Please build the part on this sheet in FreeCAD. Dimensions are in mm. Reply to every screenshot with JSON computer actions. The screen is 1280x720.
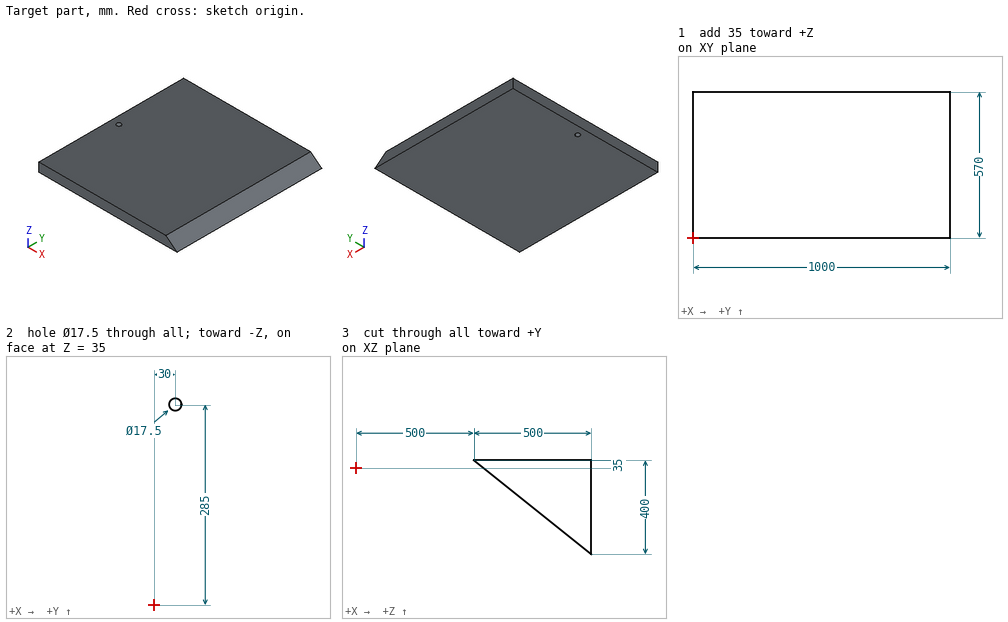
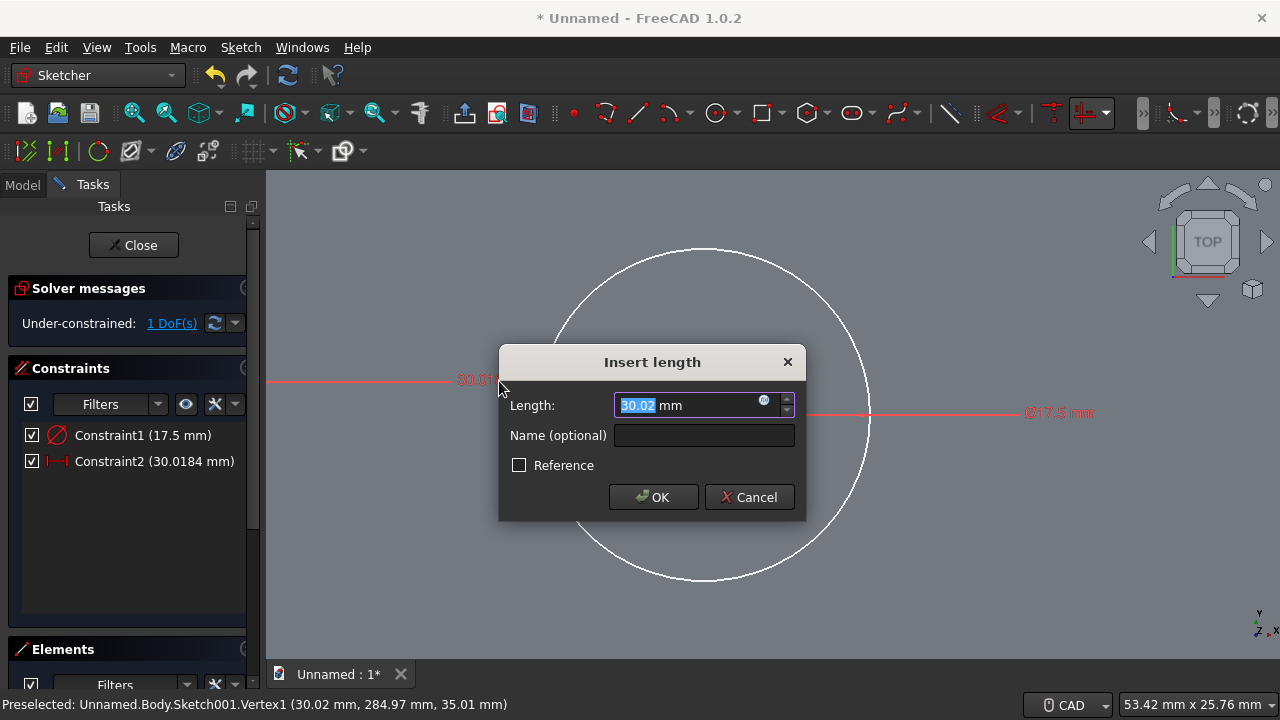
{"action": "type", "text": "30"}
{"action": "key", "text": "Return"}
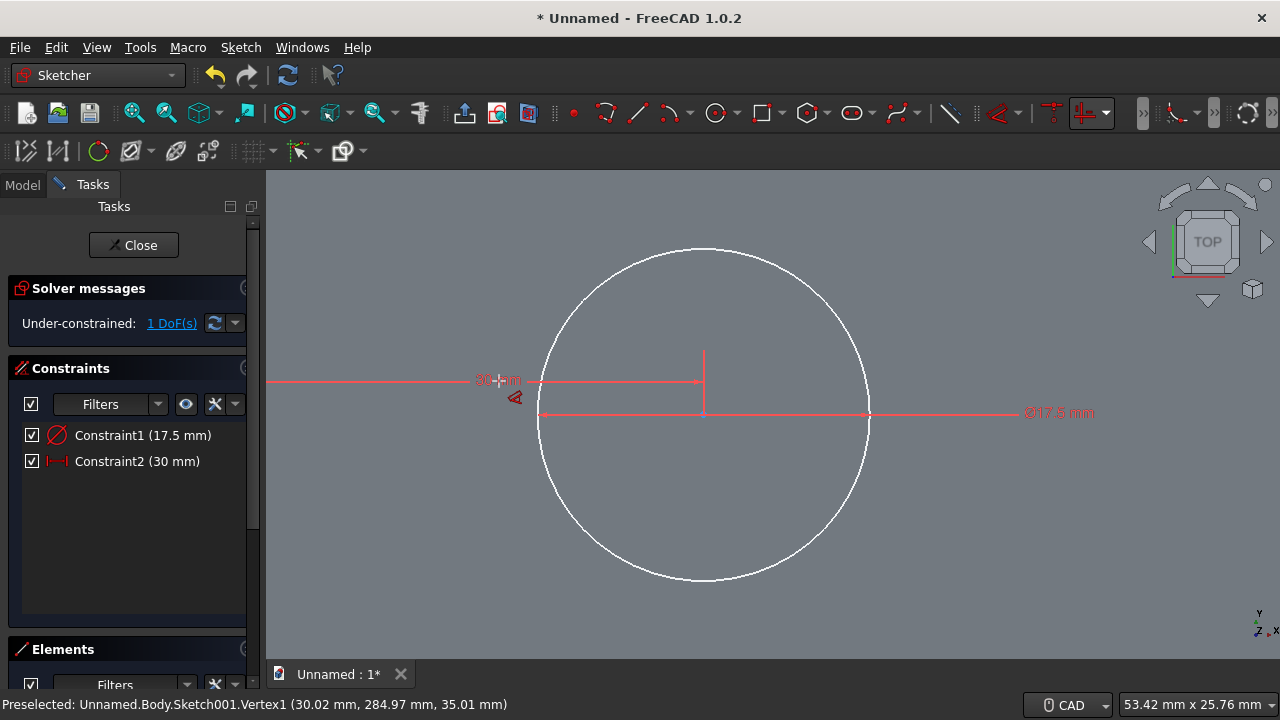
{"action": "left_click", "coordinate": [704, 415]}
{"action": "left_click", "coordinate": [738, 523]}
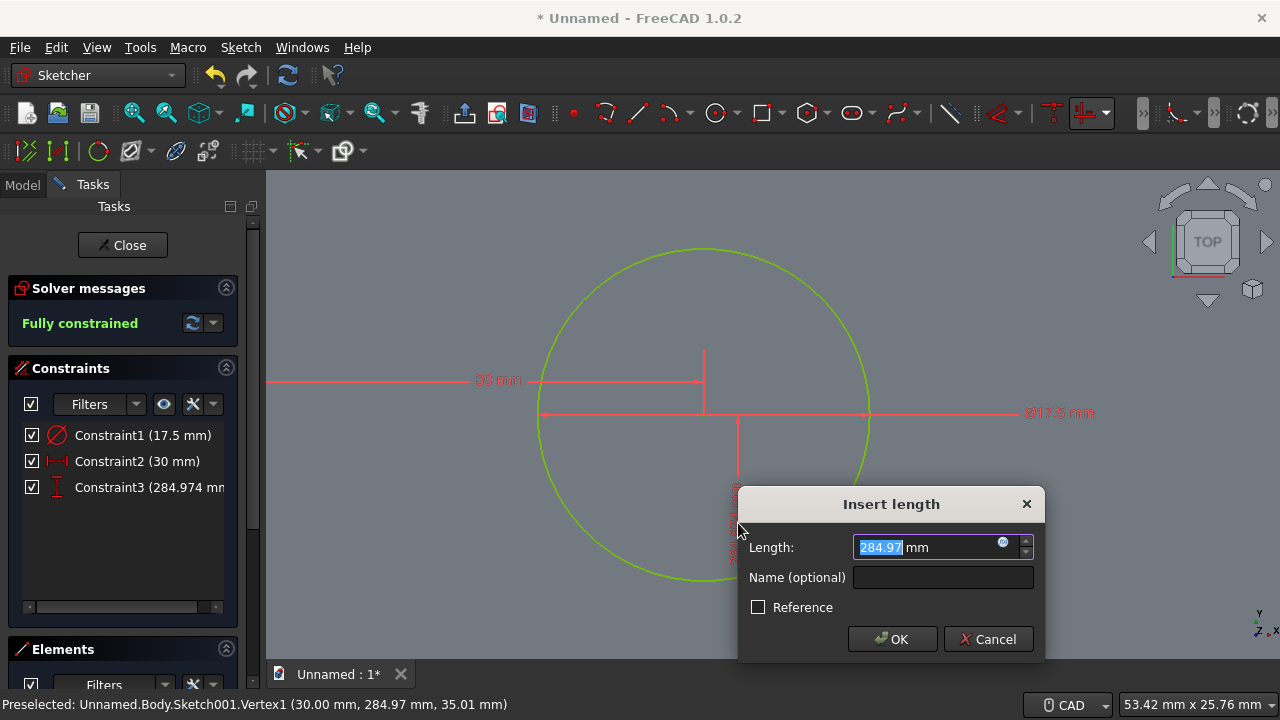
{"action": "type", "text": "285"}
{"action": "key", "text": "Return"}
{"action": "key", "text": "Escape"}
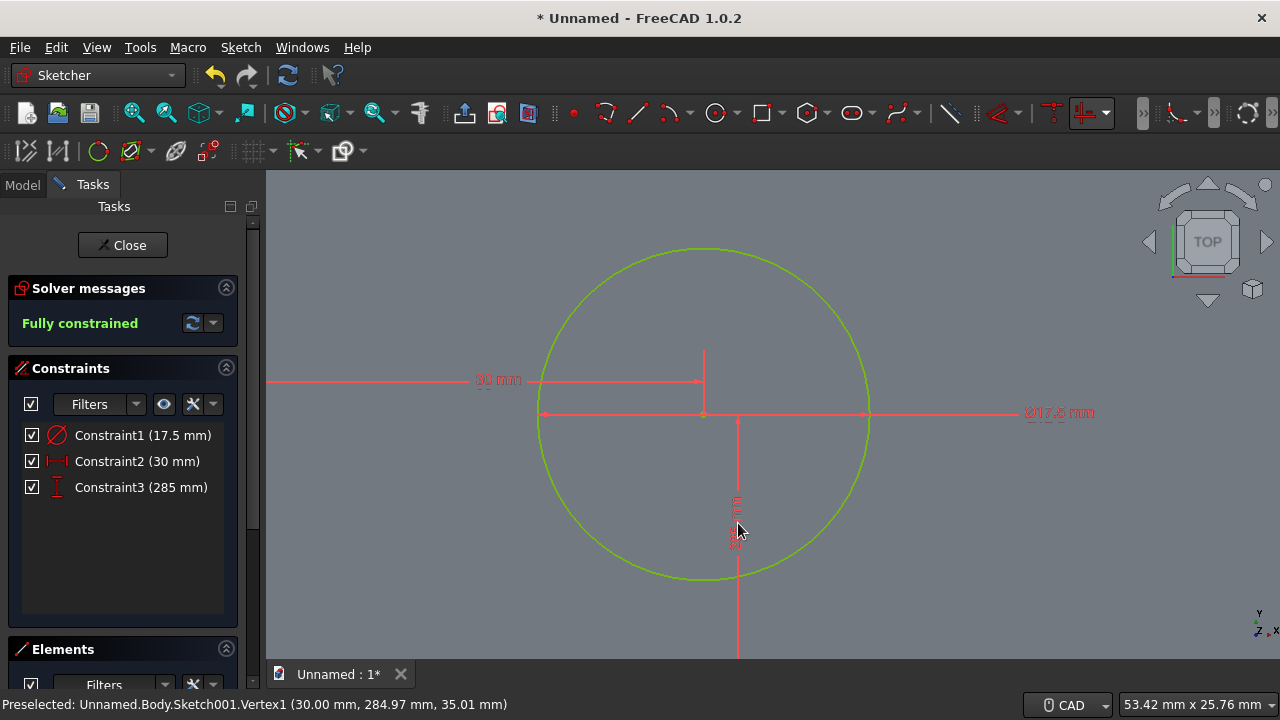
{"action": "left_click", "coordinate": [123, 245]}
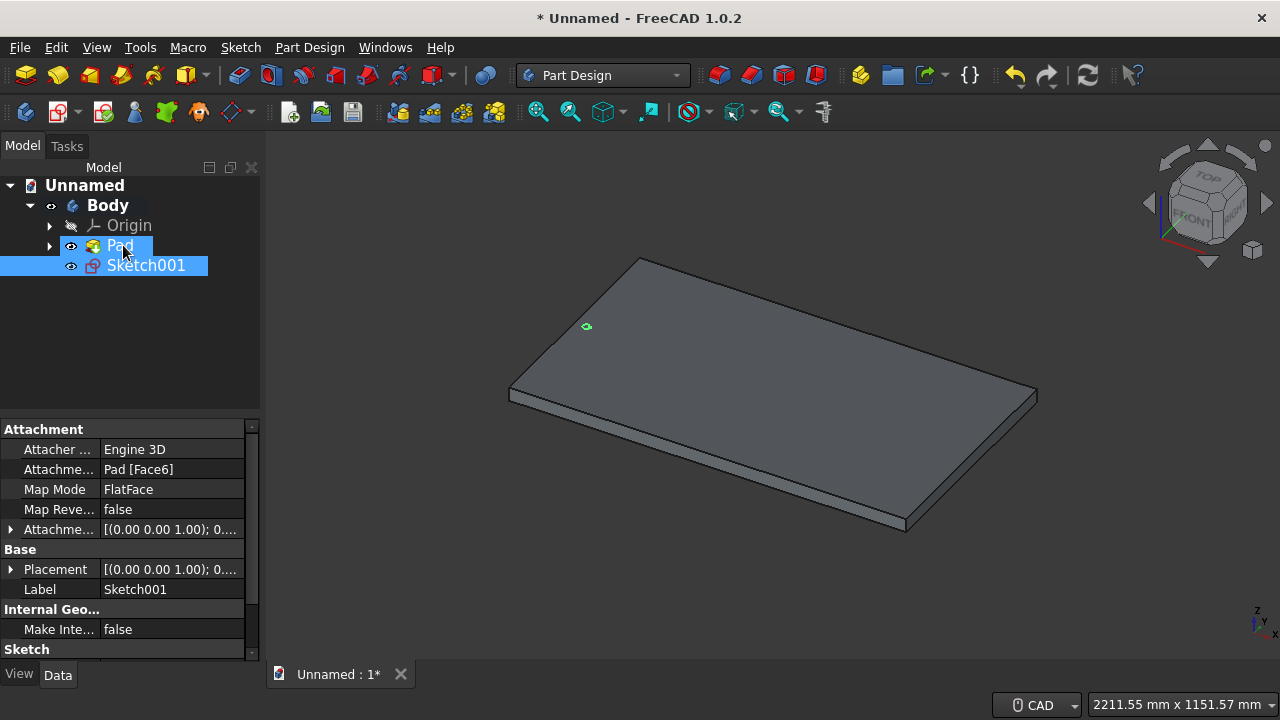
{"action": "left_click", "coordinate": [272, 76]}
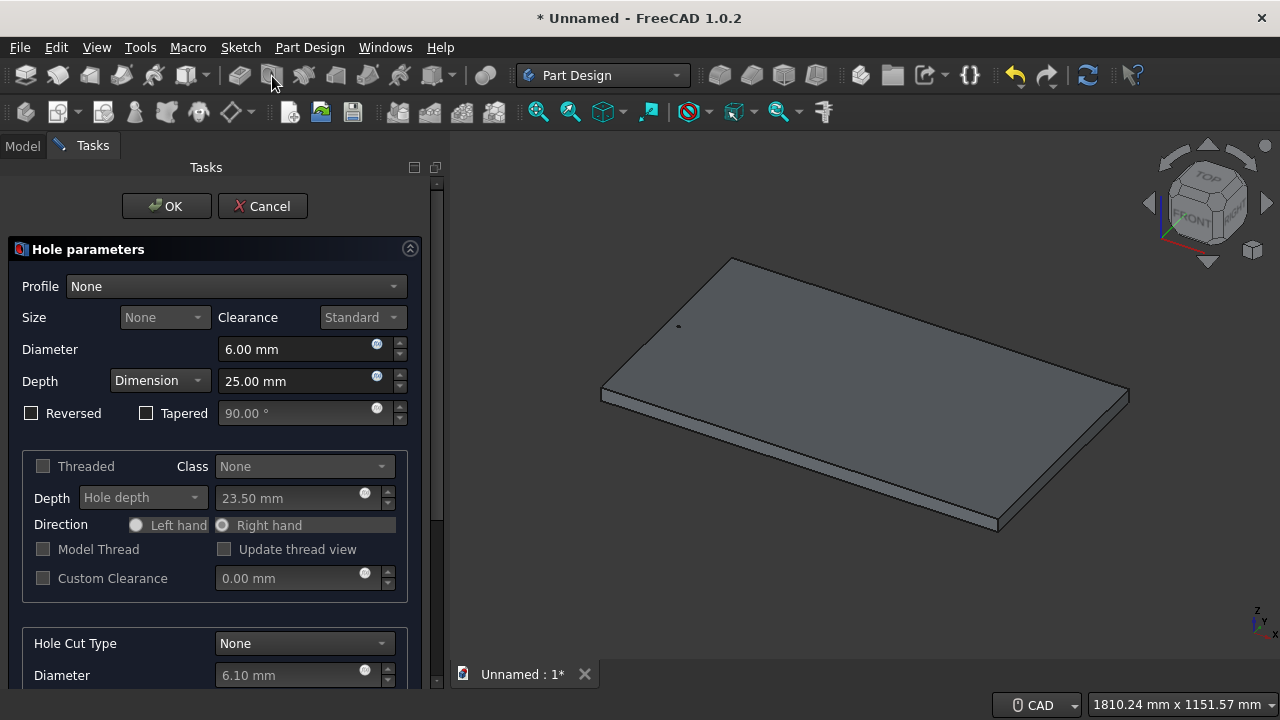
{"action": "triple_click", "coordinate": [305, 349]}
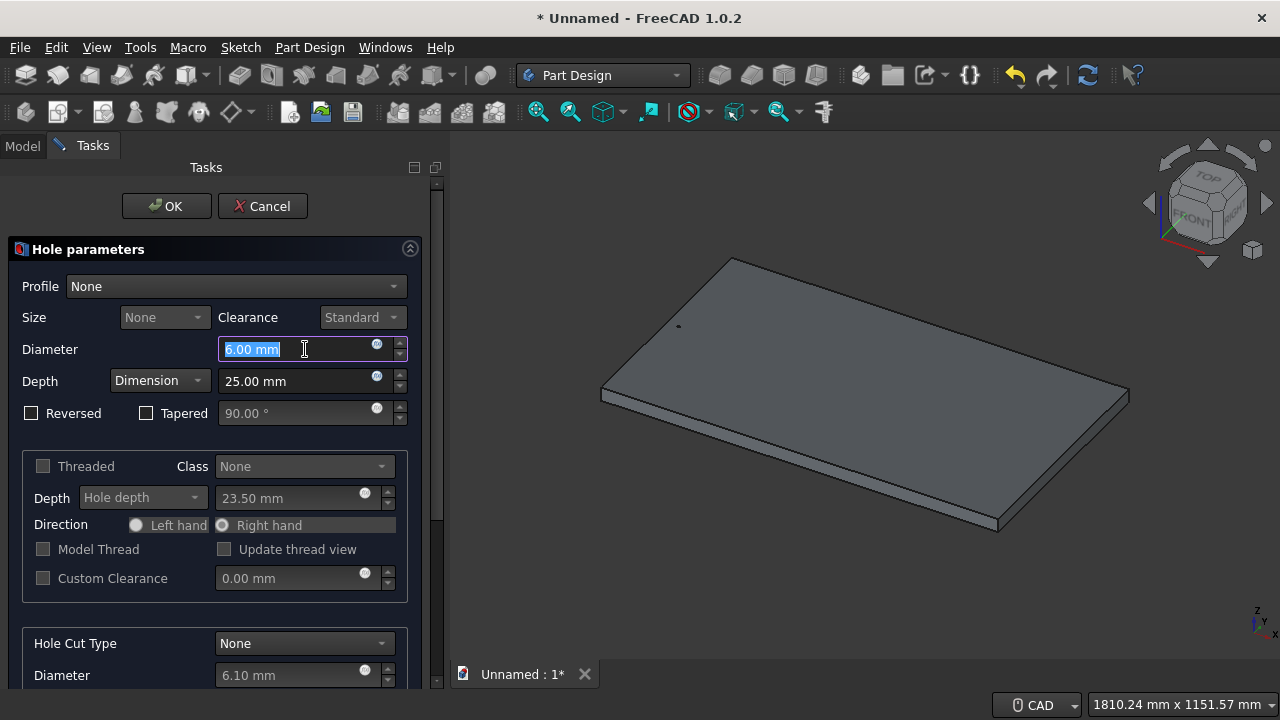
{"action": "type", "text": "17.5"}
{"action": "key", "text": "Tab"}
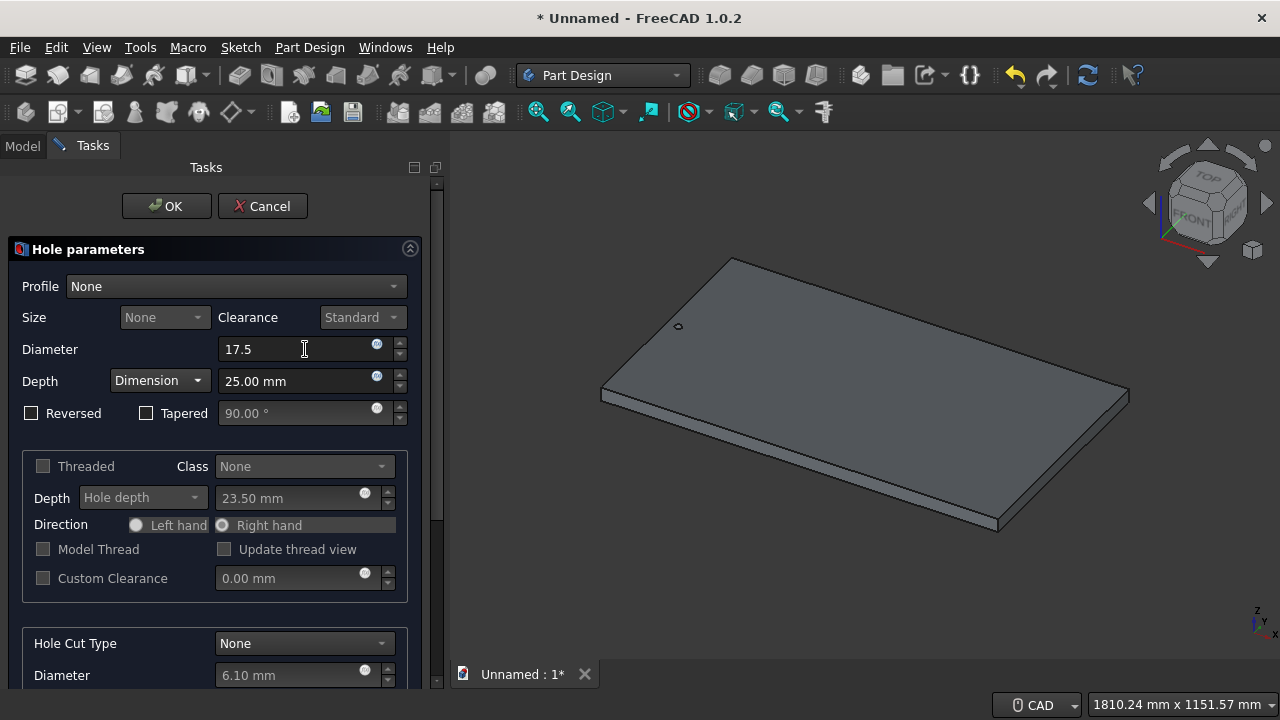
{"action": "left_click", "coordinate": [161, 380]}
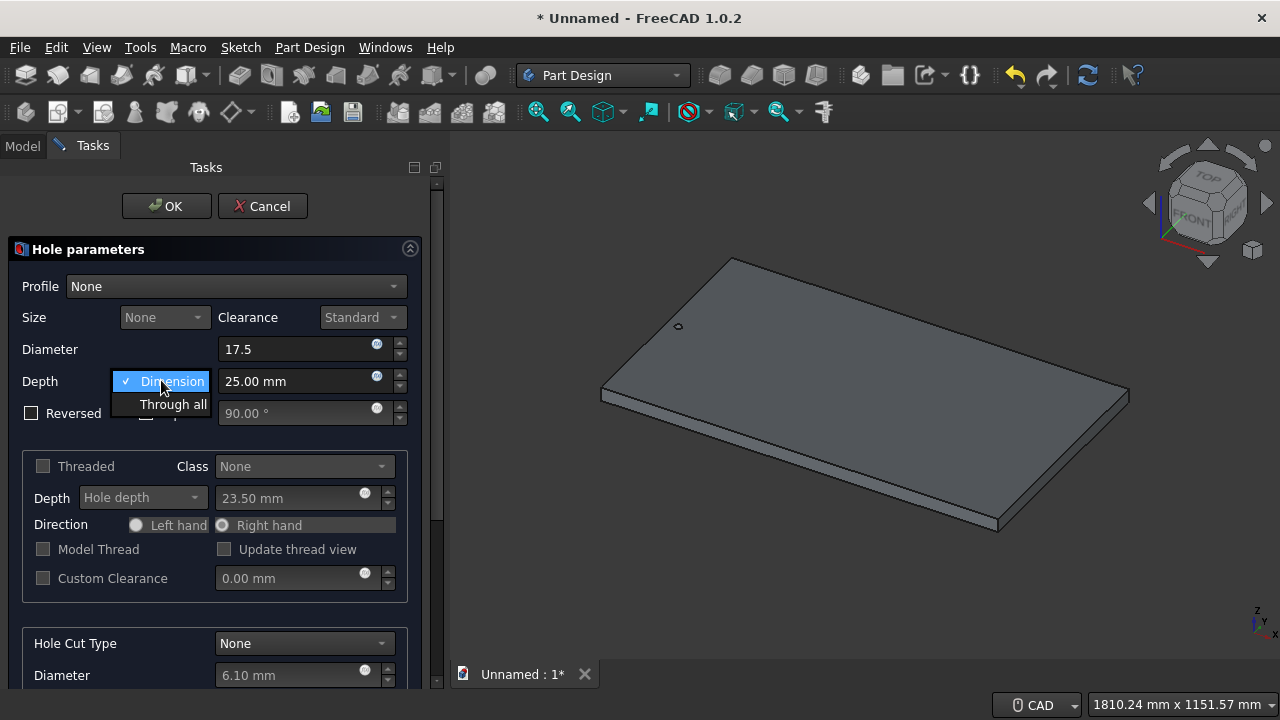
{"action": "left_click", "coordinate": [160, 404]}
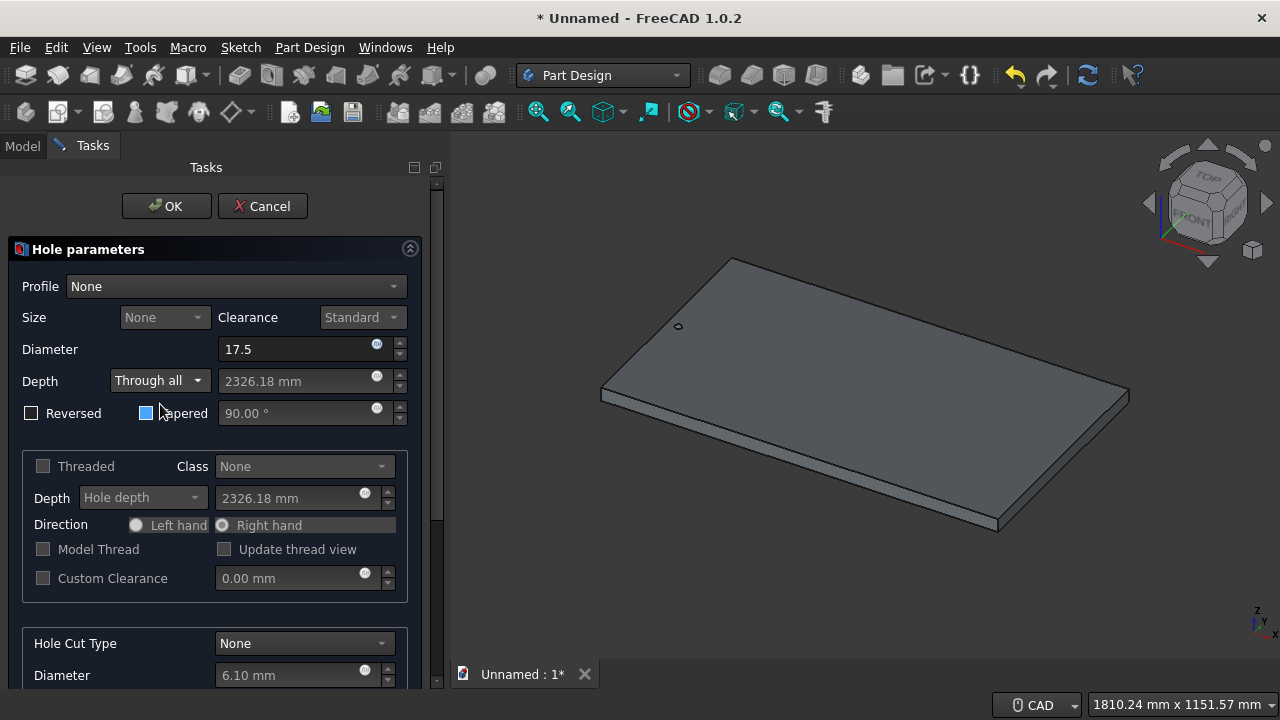
{"action": "left_click", "coordinate": [167, 206]}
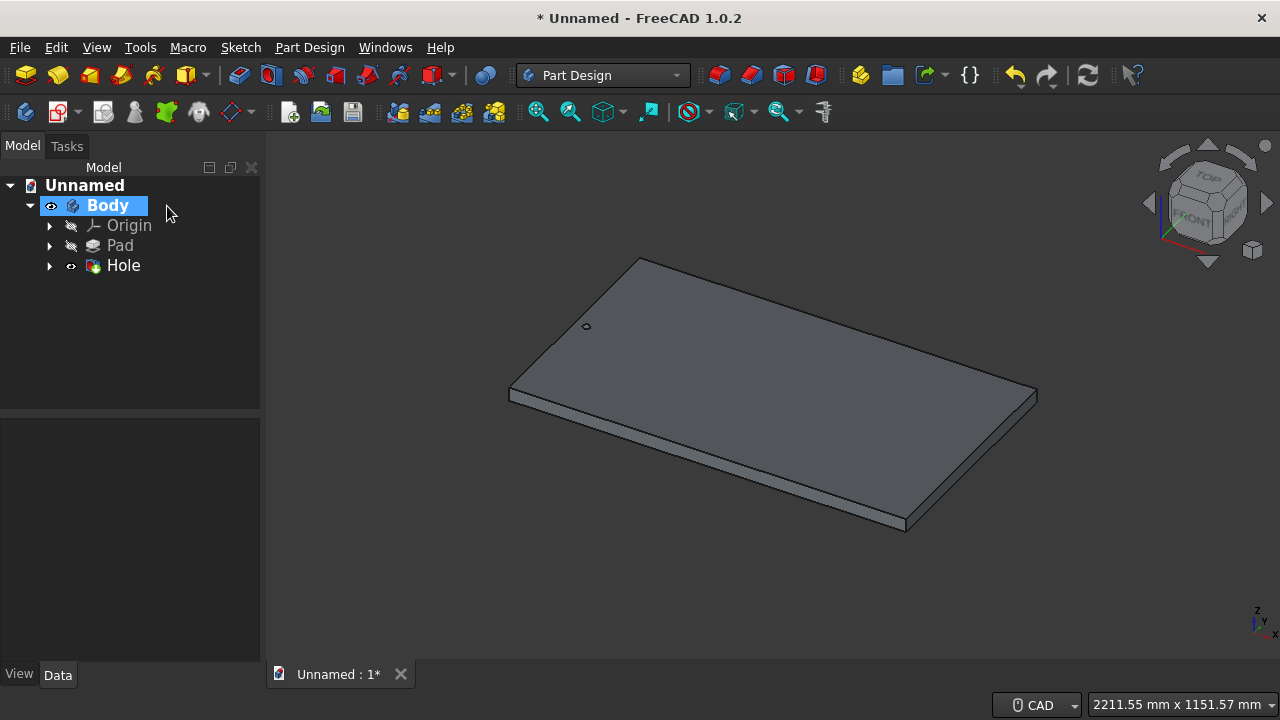
{"action": "left_click", "coordinate": [58, 112]}